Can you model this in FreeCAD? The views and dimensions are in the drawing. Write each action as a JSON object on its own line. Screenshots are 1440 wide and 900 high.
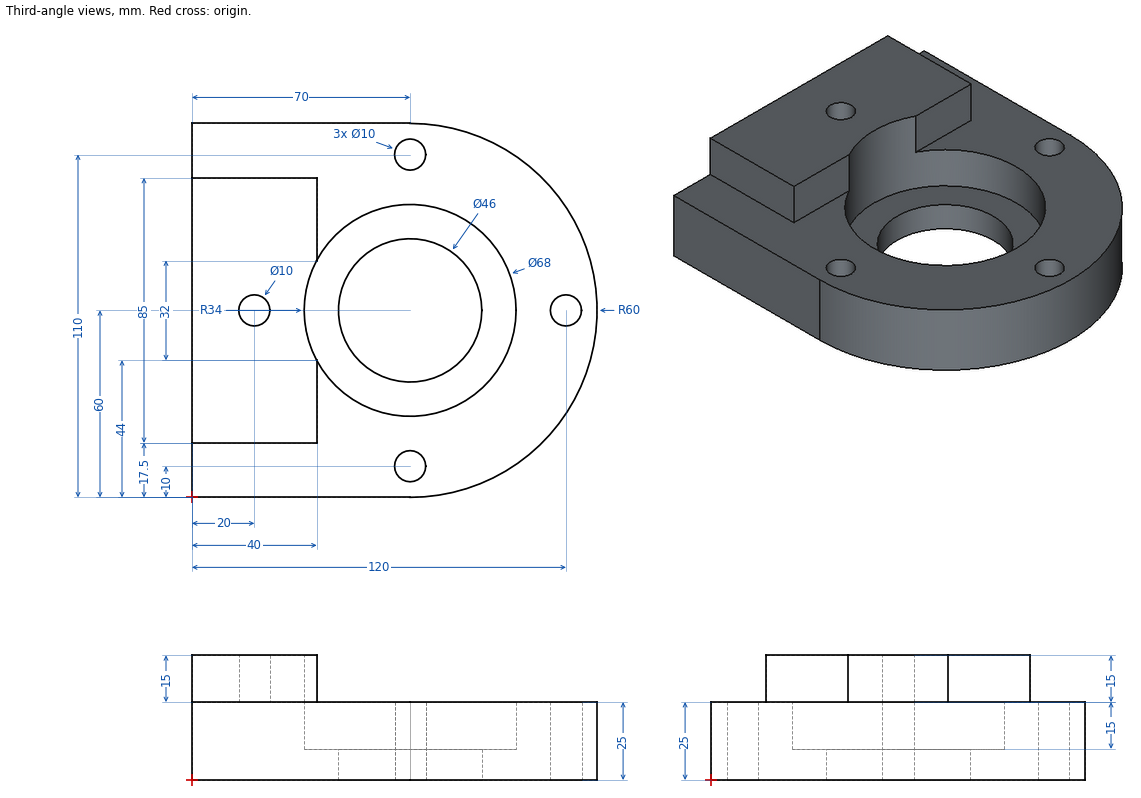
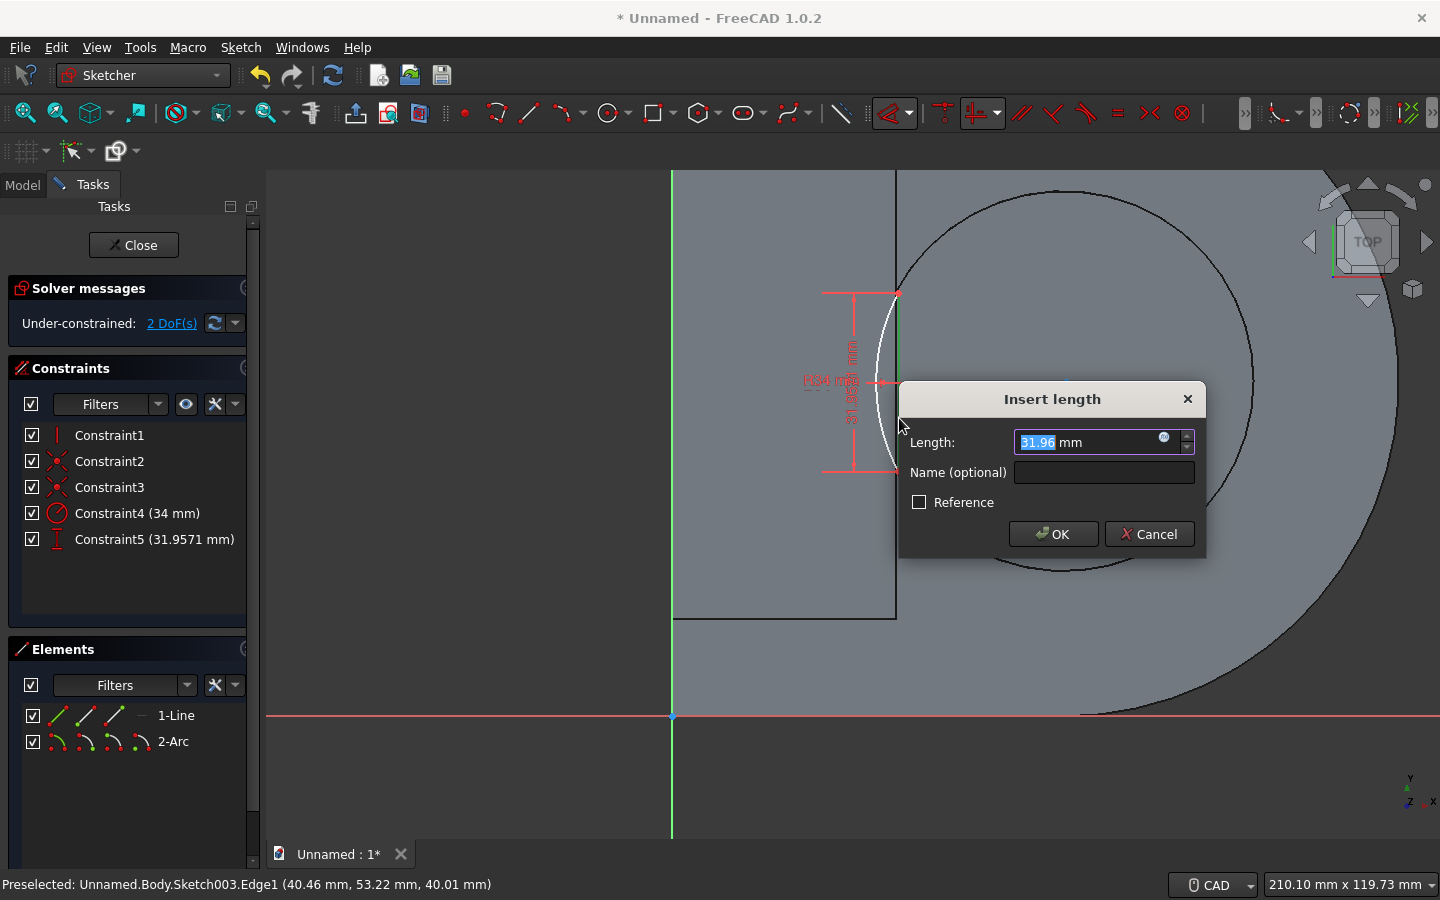
{"action": "type", "text": "32"}
{"action": "key", "text": "Return"}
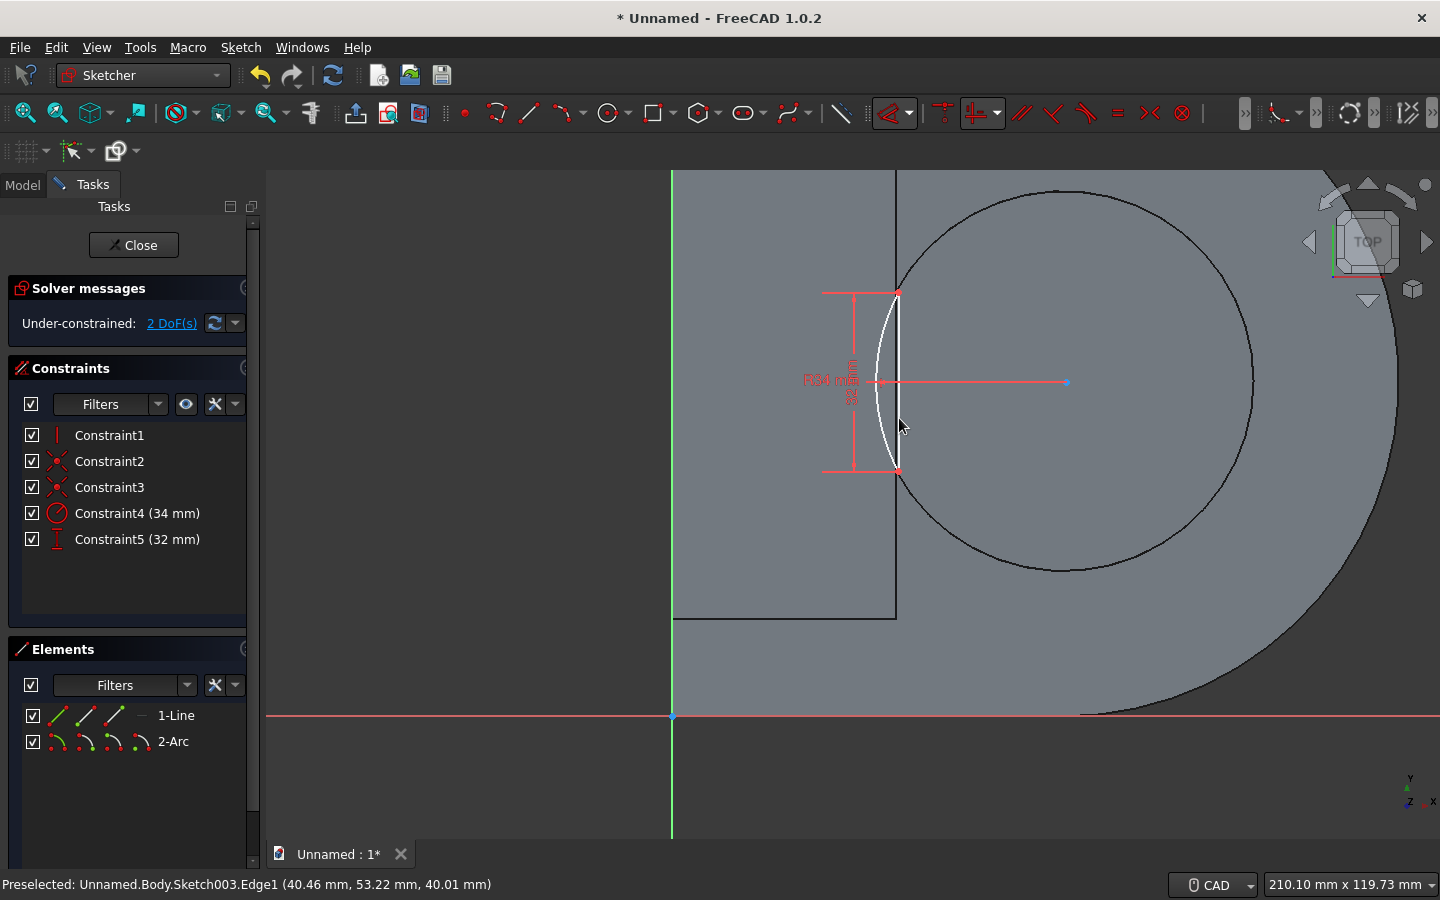
{"action": "left_click", "coordinate": [899, 472]}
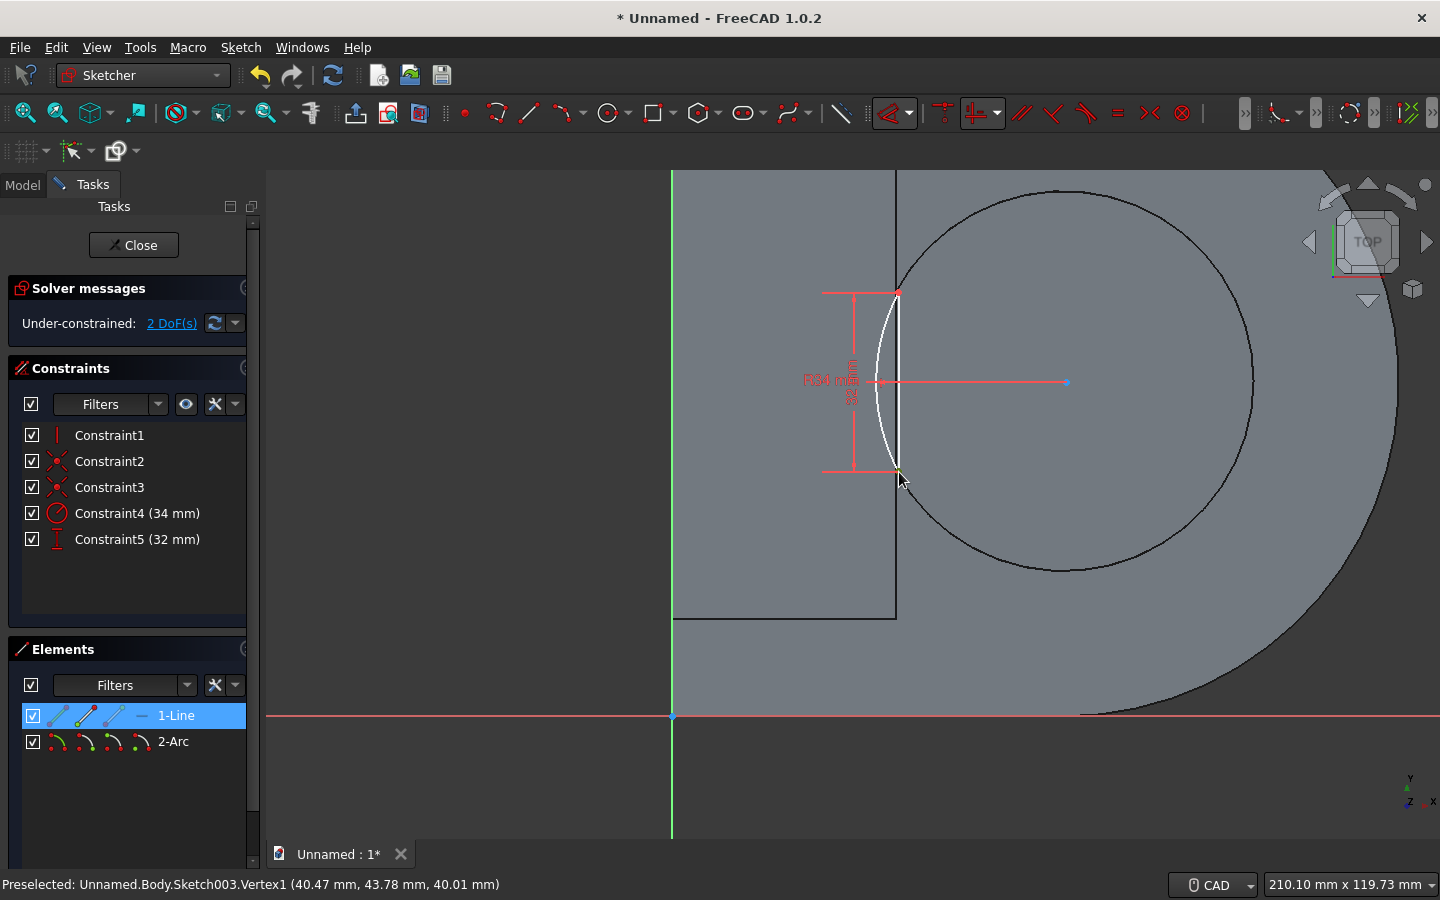
{"action": "left_click", "coordinate": [912, 114]}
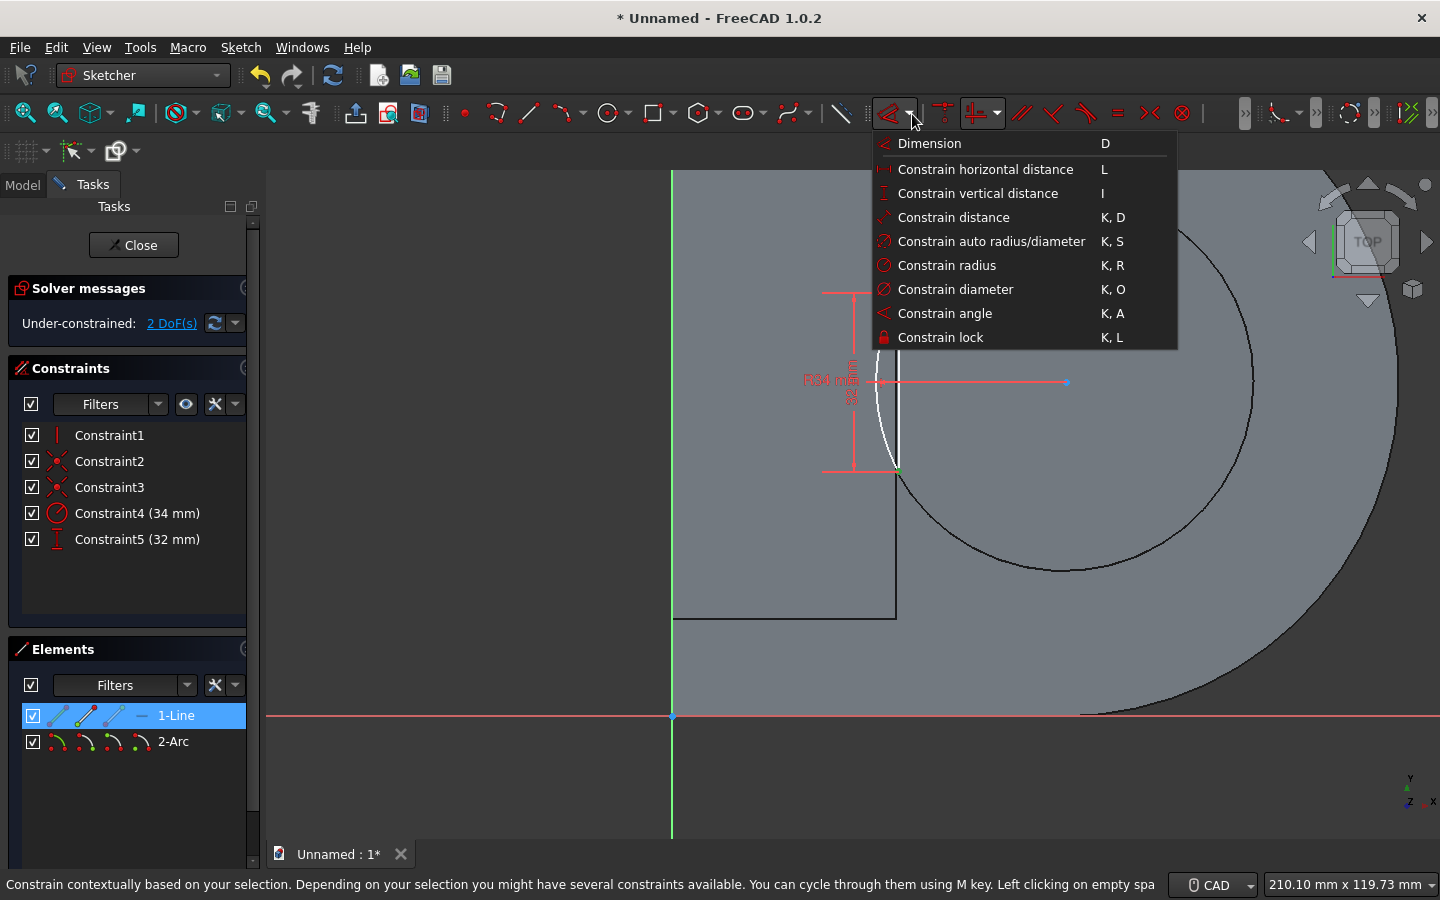
{"action": "left_click", "coordinate": [1025, 169]}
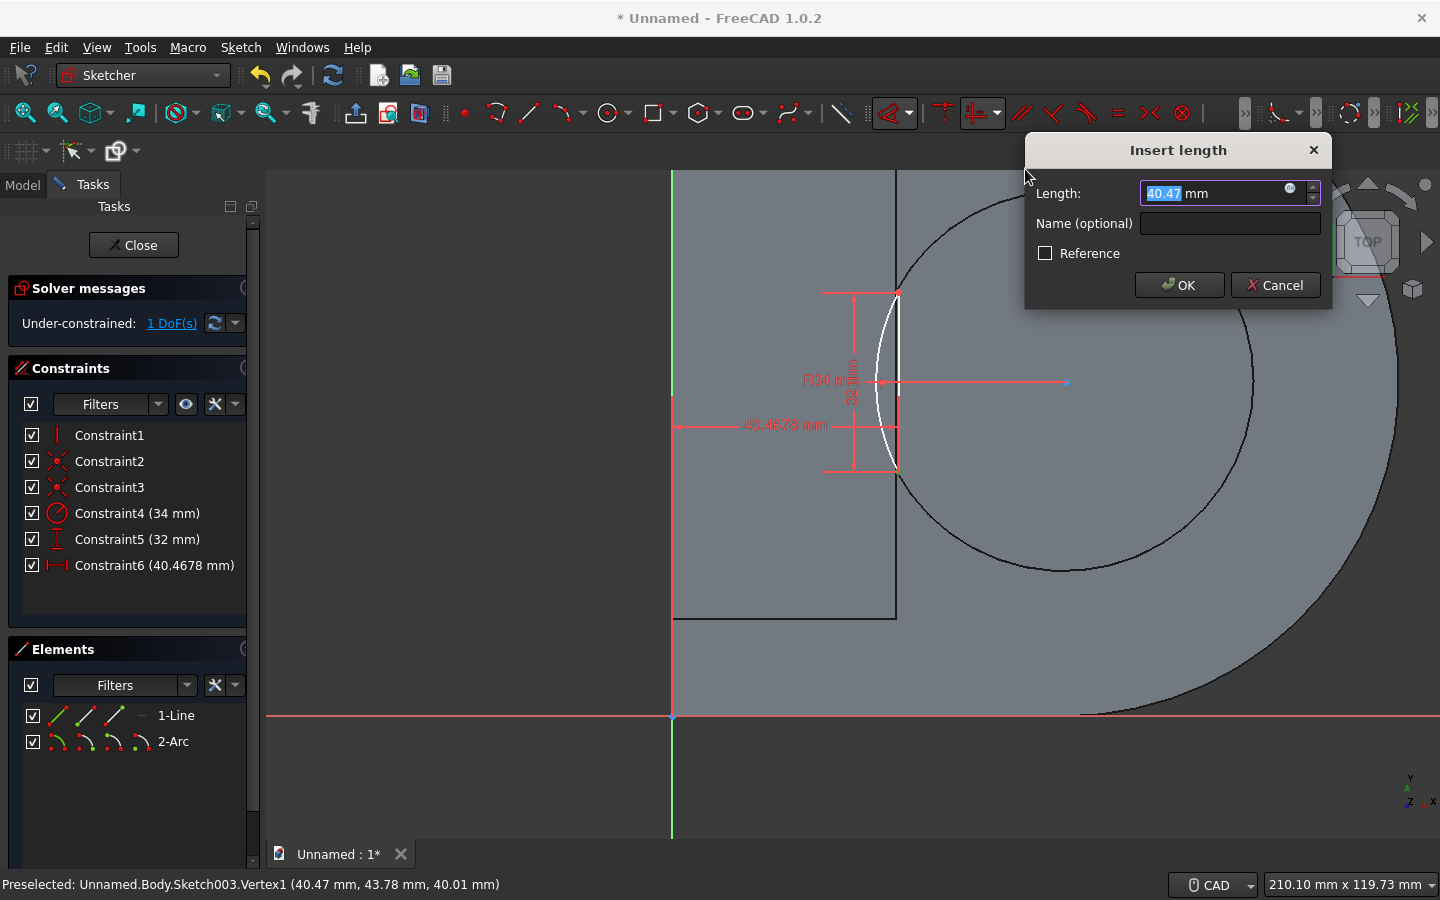
{"action": "type", "text": "40"}
{"action": "key", "text": "Return"}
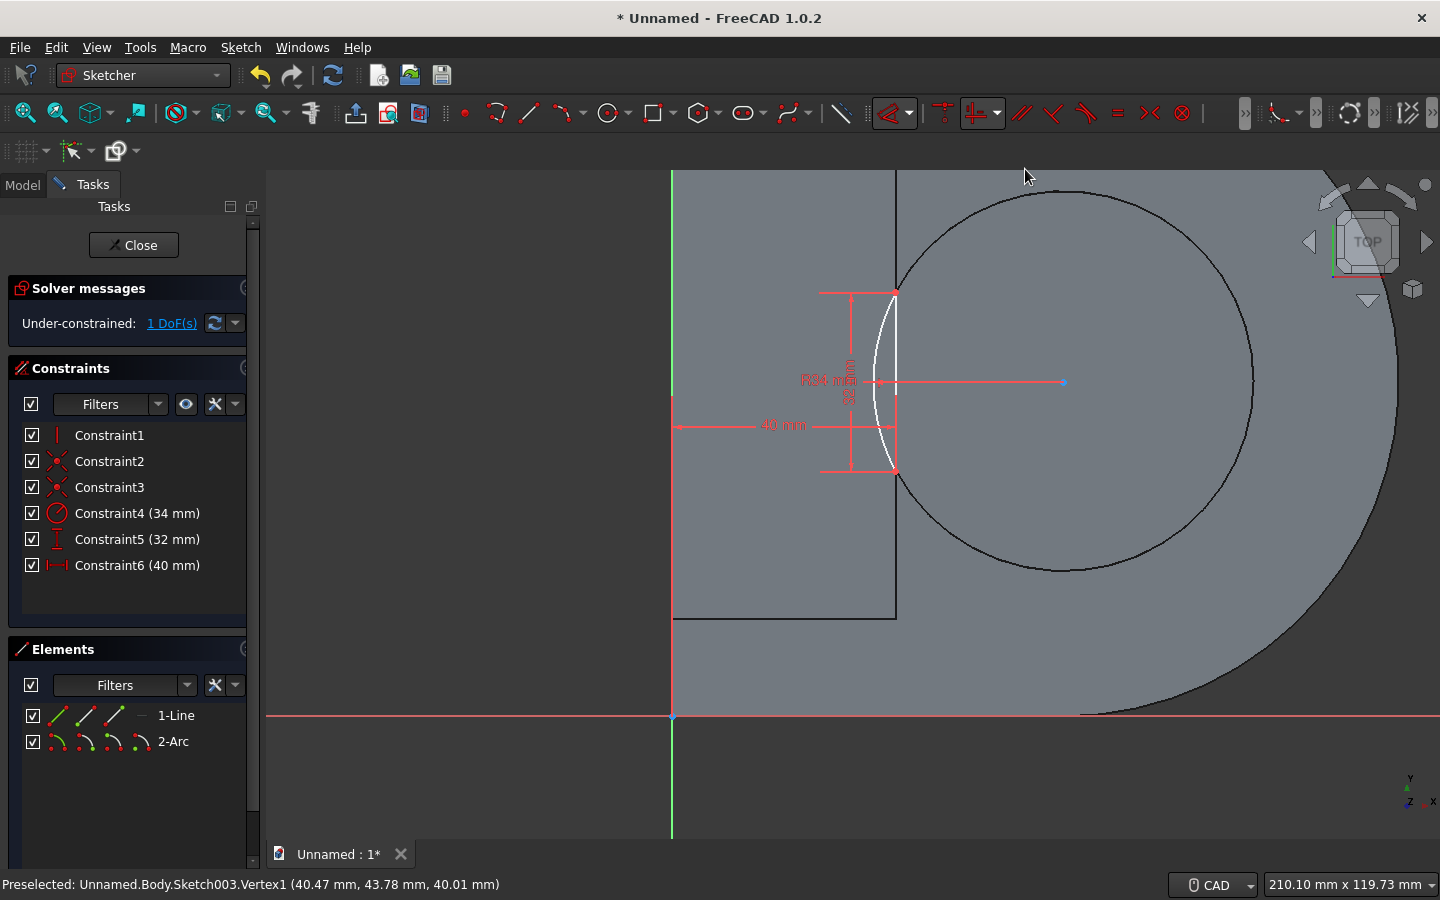
{"action": "left_click", "coordinate": [896, 472]}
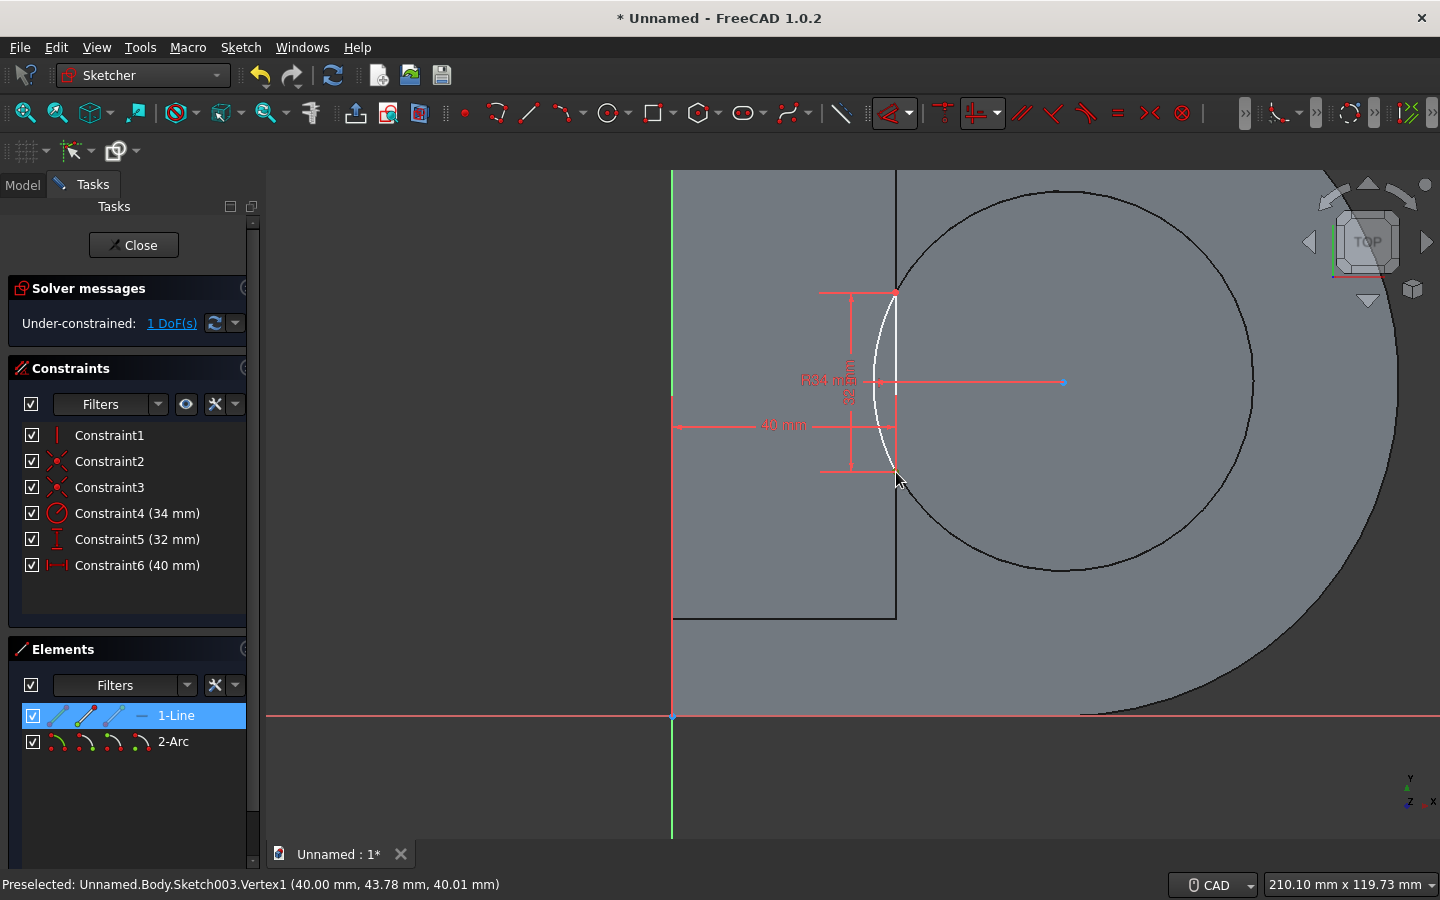
{"action": "left_click", "coordinate": [912, 114]}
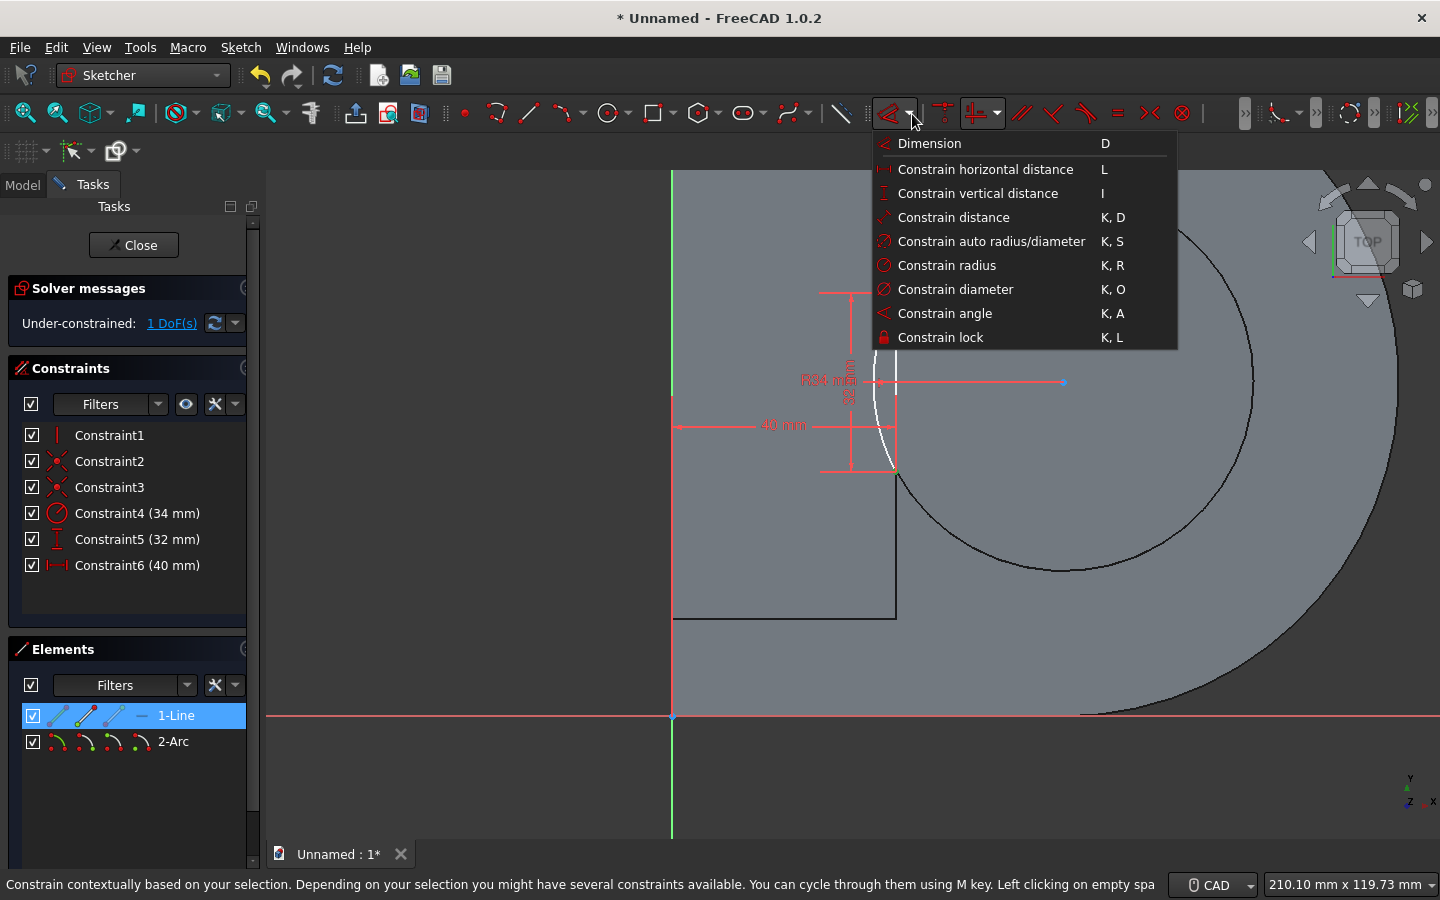
{"action": "left_click", "coordinate": [1025, 193]}